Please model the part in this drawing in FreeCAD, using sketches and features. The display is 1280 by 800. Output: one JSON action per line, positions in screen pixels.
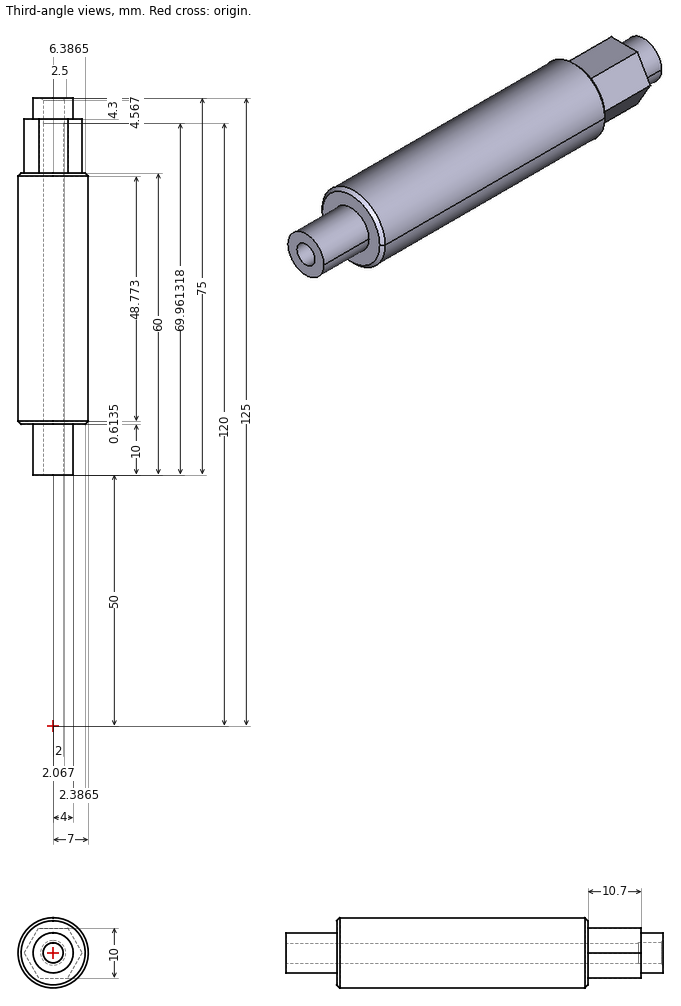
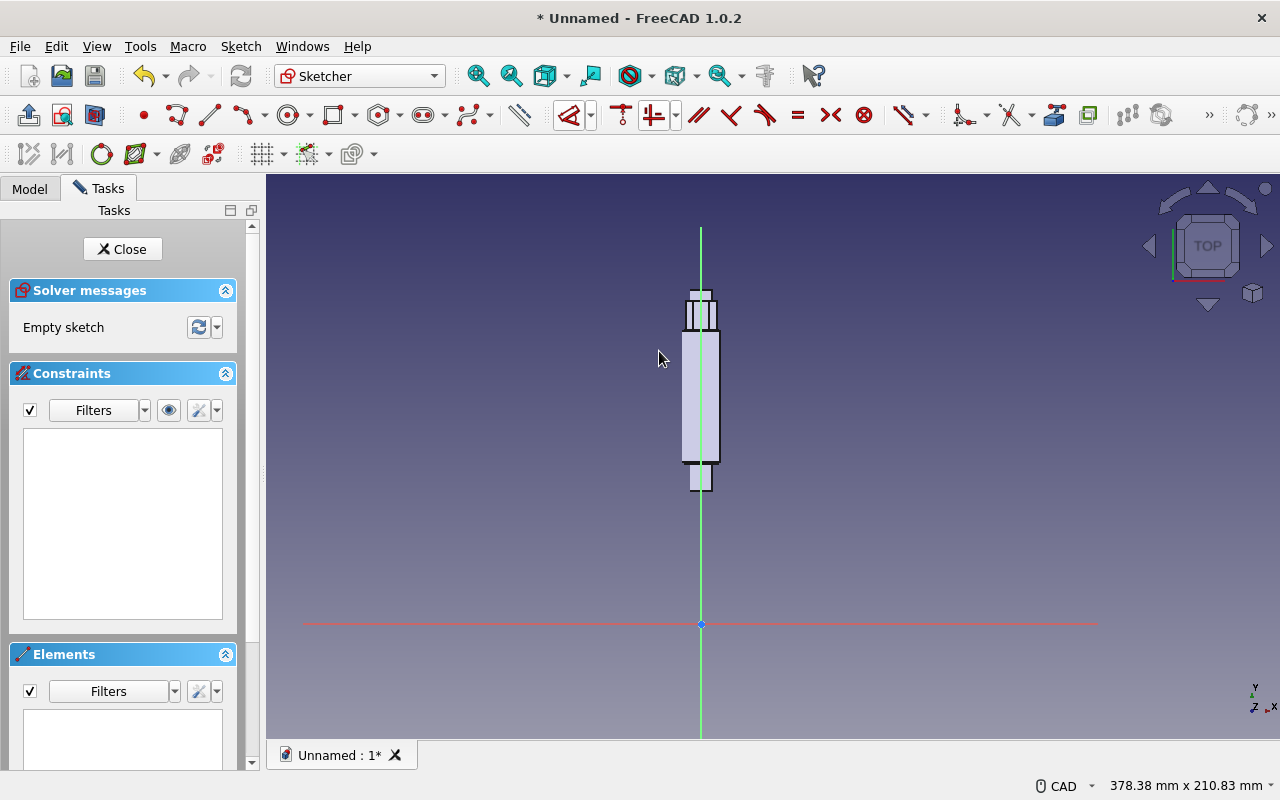
{"action": "left_click", "coordinate": [177, 116]}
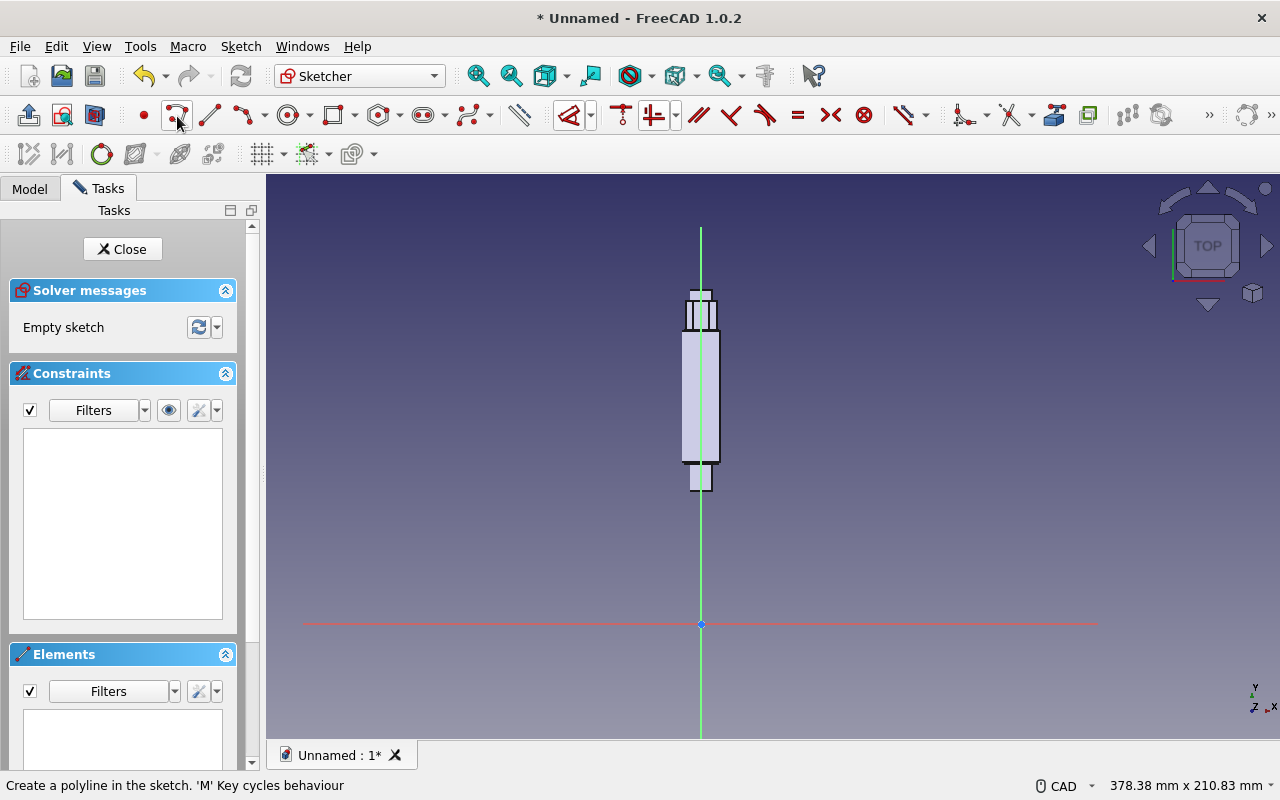
{"action": "left_click", "coordinate": [701, 491]}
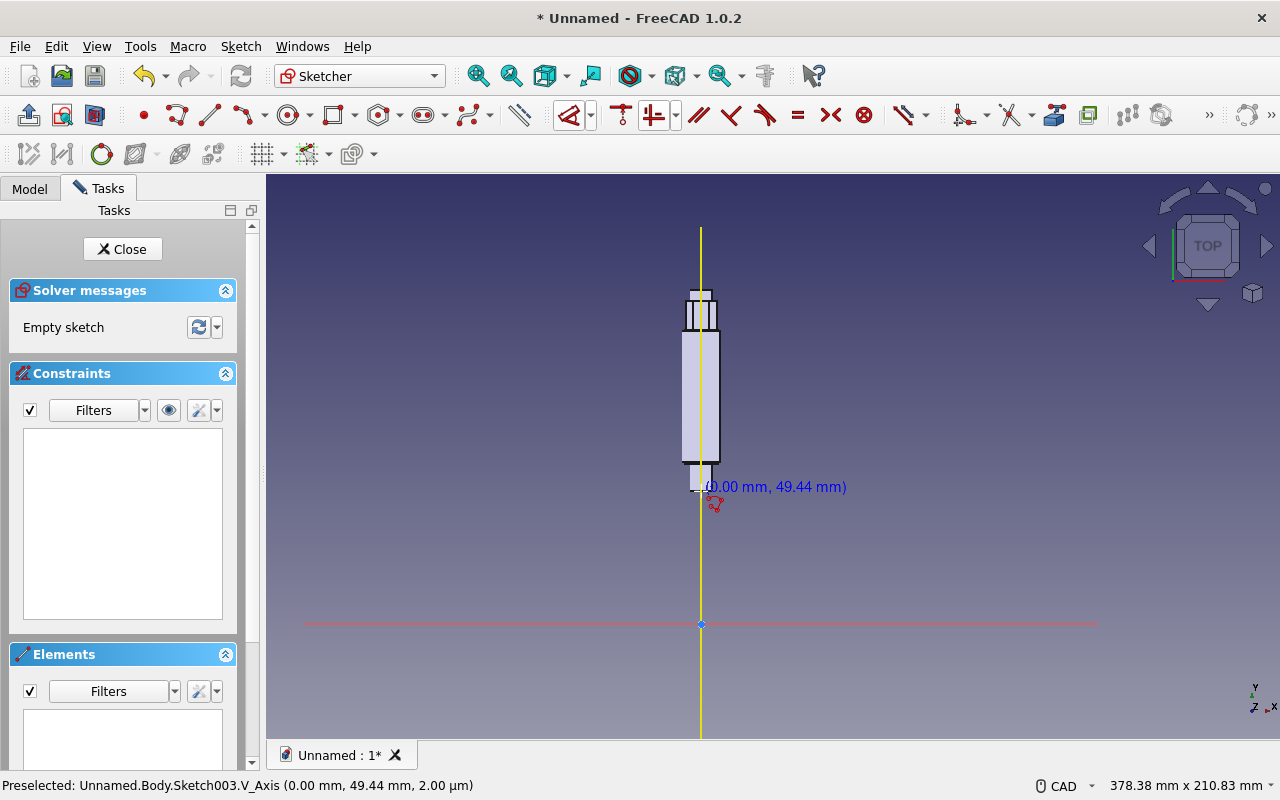
{"action": "scroll", "coordinate": [707, 491], "scroll_direction": "up", "scroll_amount": 6}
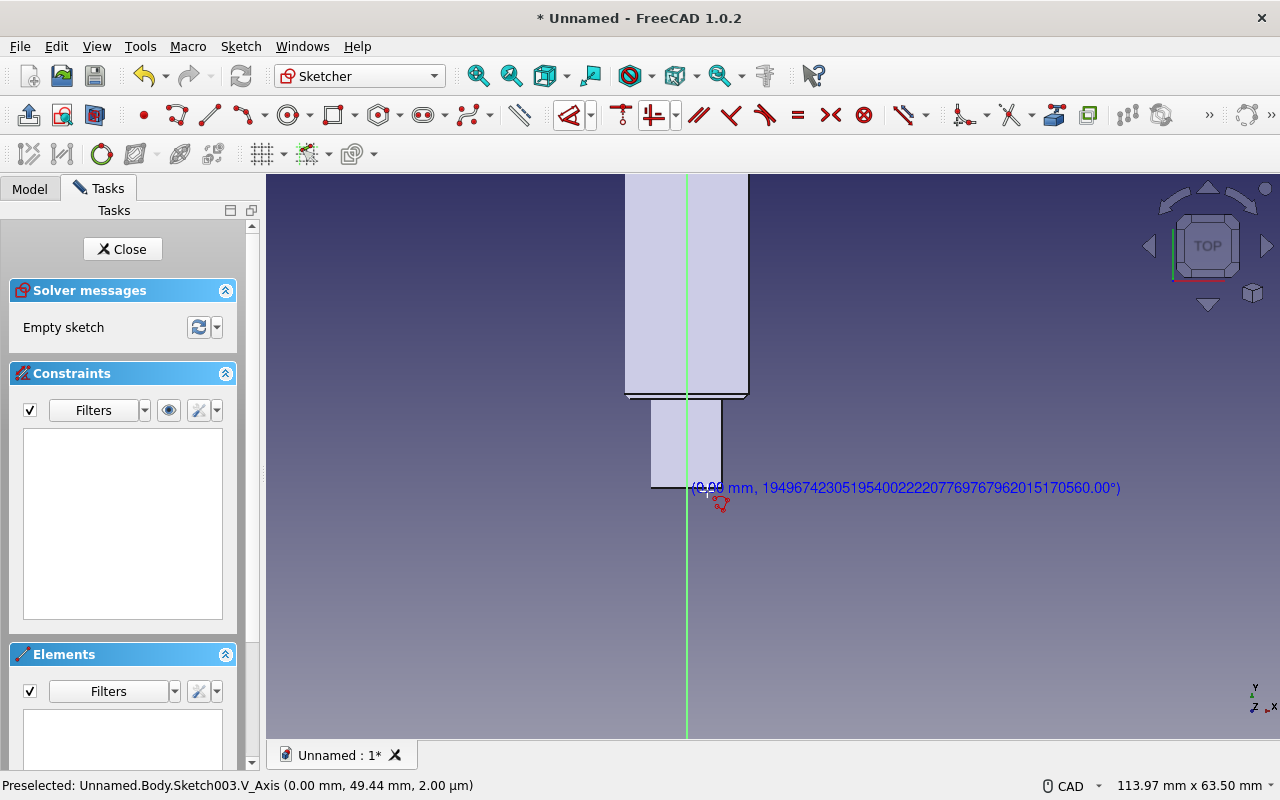
{"action": "left_click", "coordinate": [704, 490]}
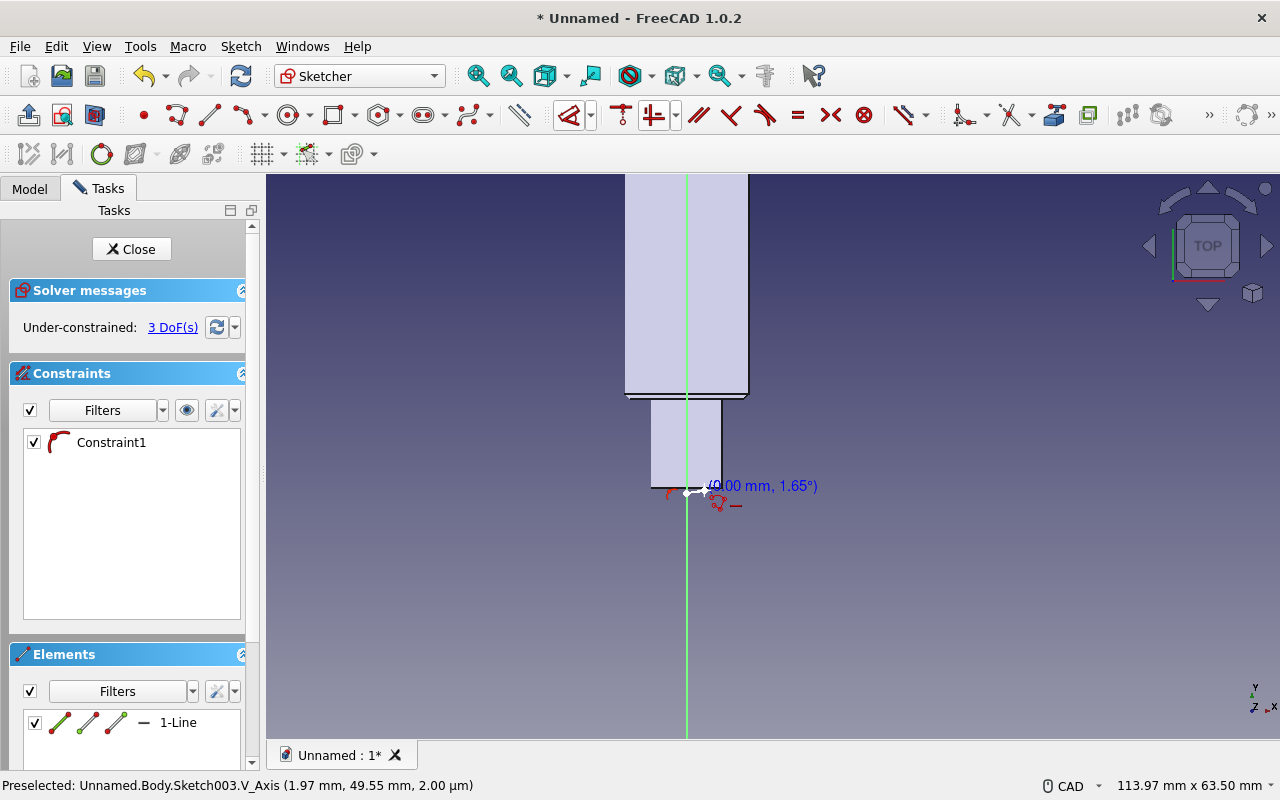
{"action": "scroll", "coordinate": [707, 491], "scroll_direction": "down", "scroll_amount": 6}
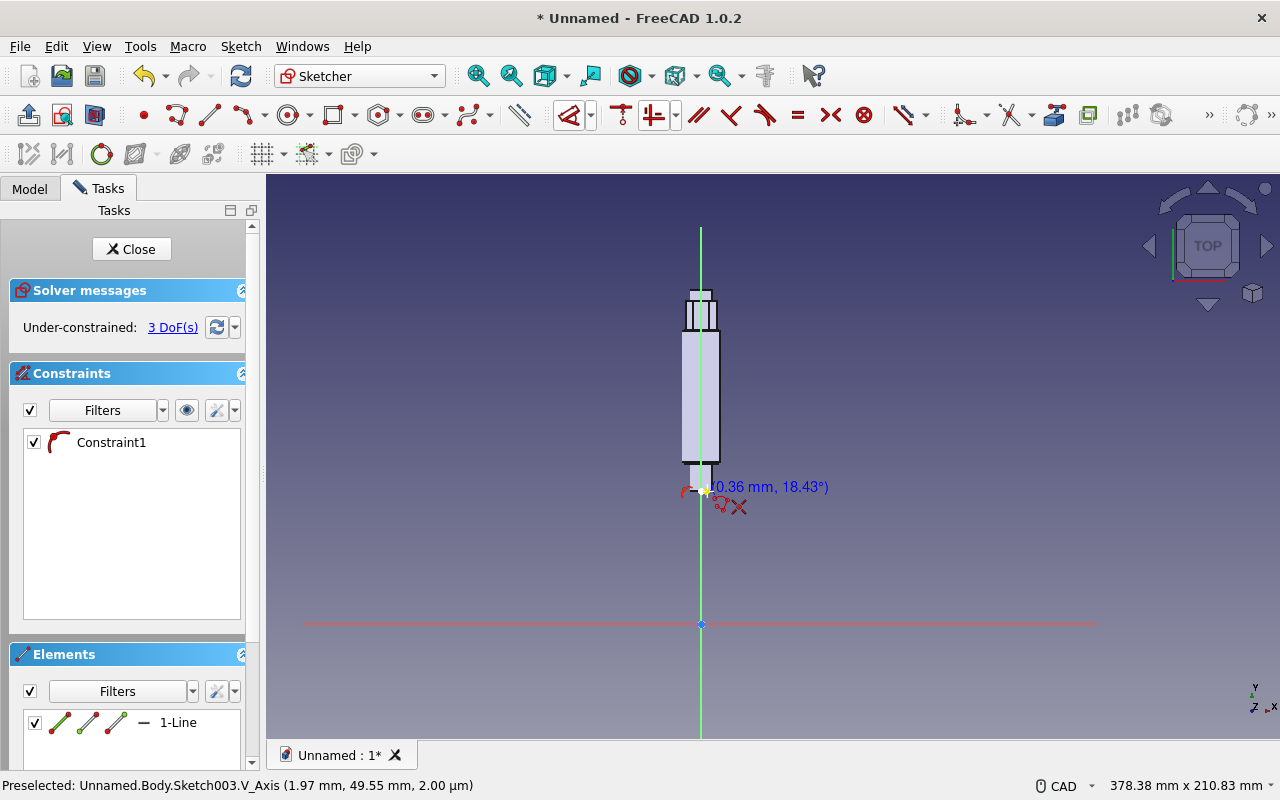
{"action": "scroll", "coordinate": [707, 303], "scroll_direction": "up", "scroll_amount": 6}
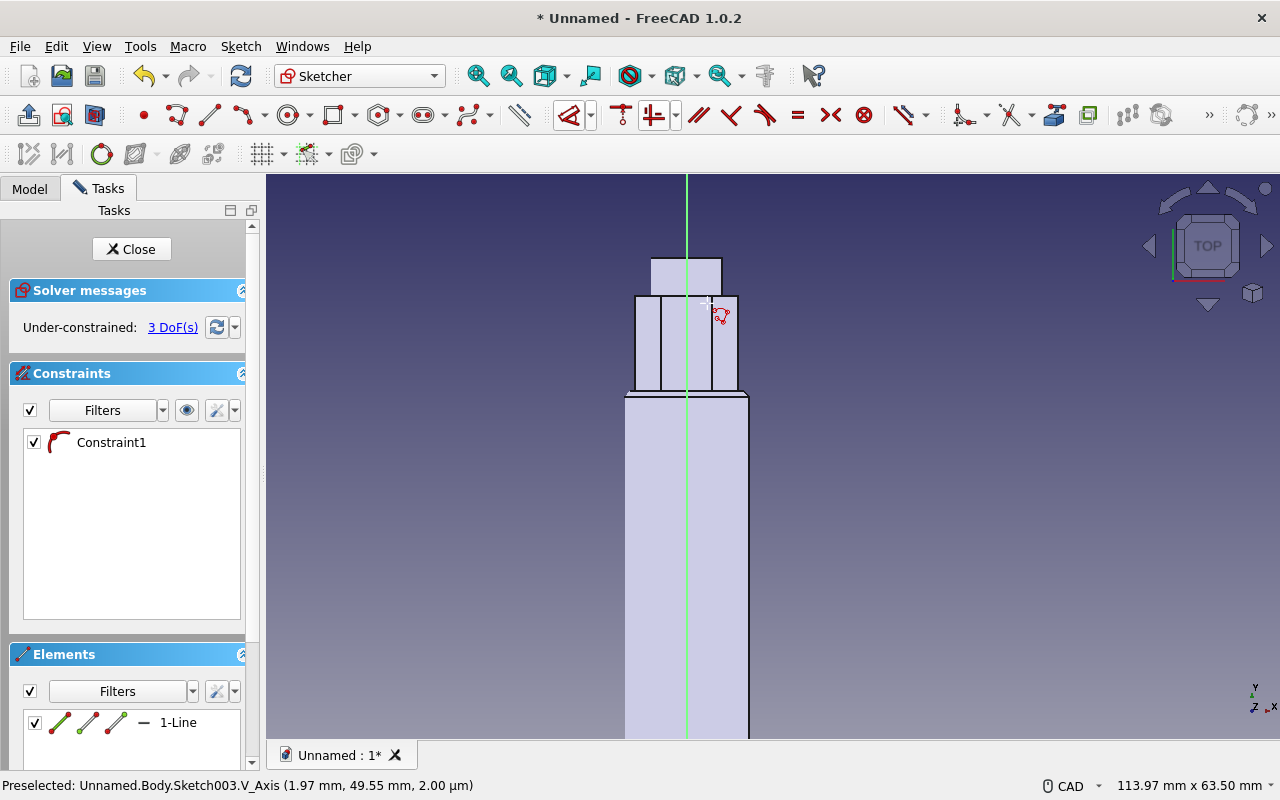
{"action": "left_click", "coordinate": [704, 303]}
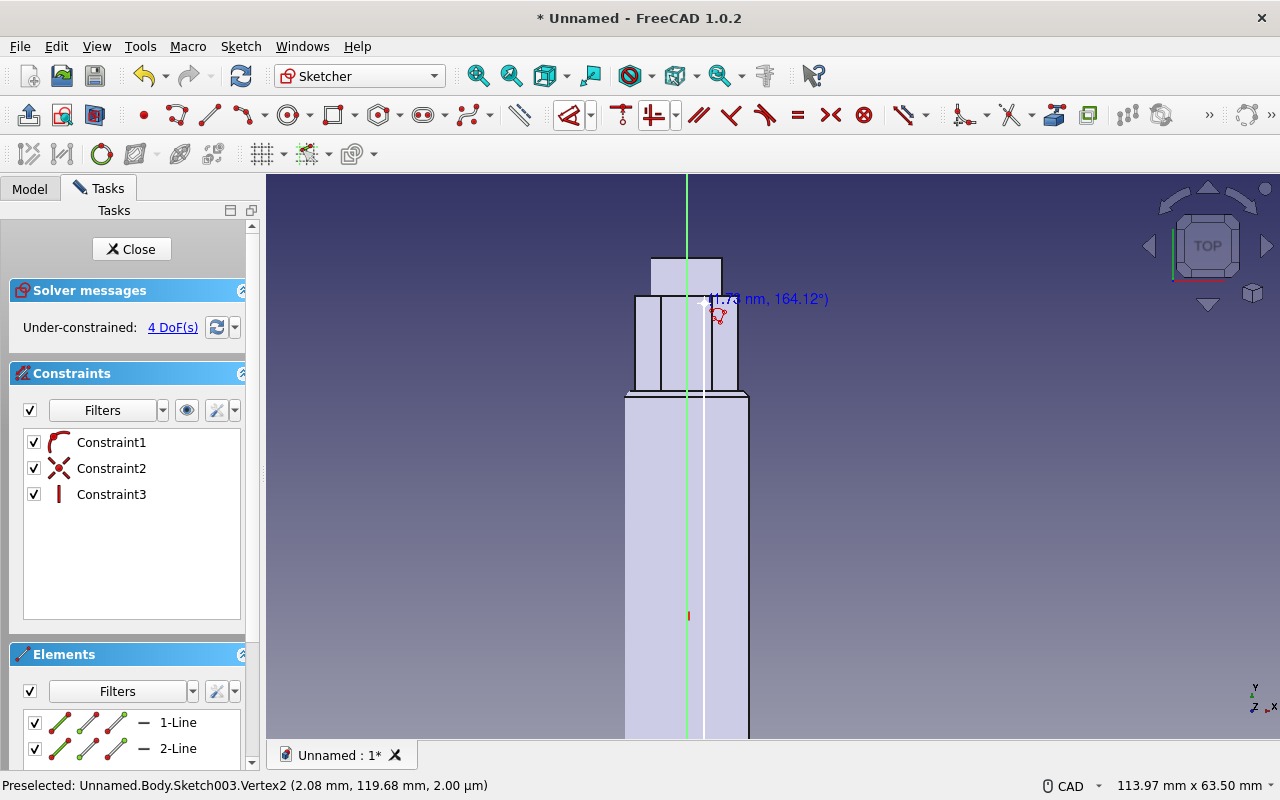
{"action": "scroll", "coordinate": [705, 302], "scroll_direction": "up", "scroll_amount": 16}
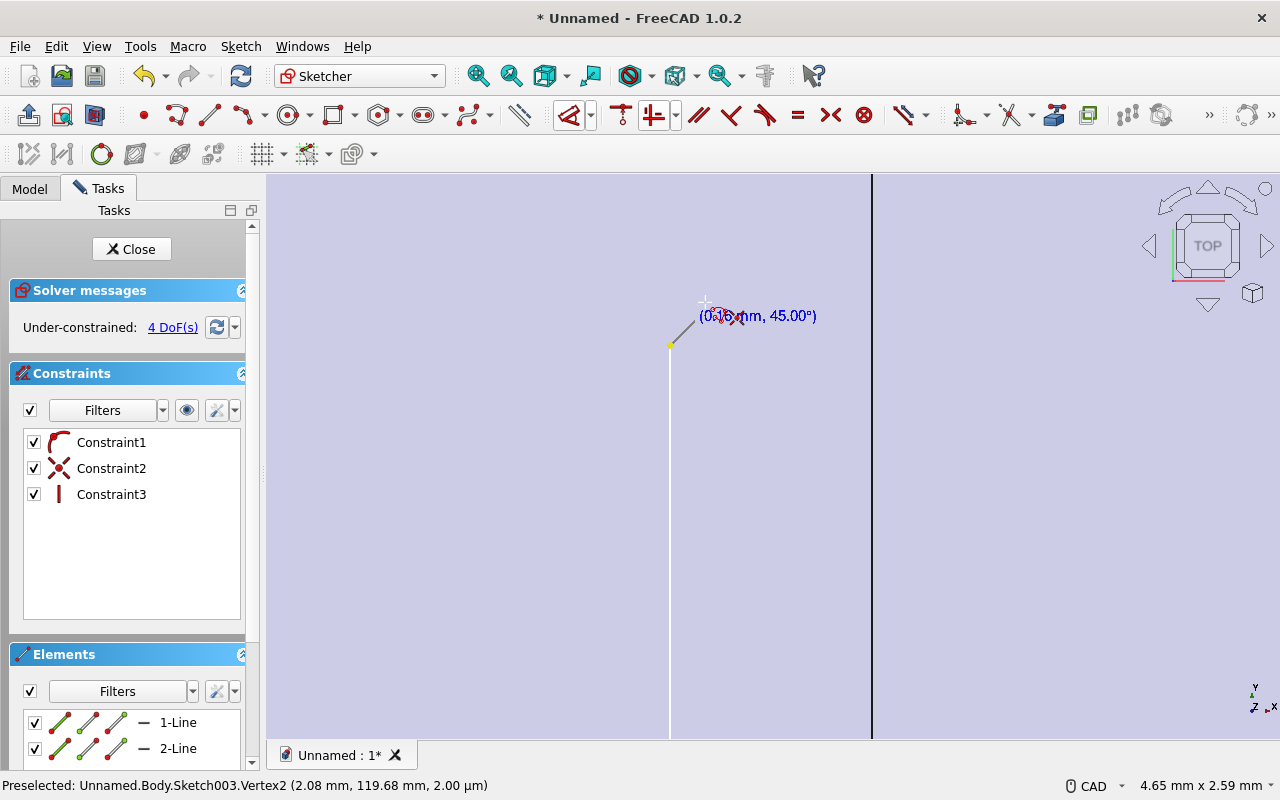
{"action": "left_click", "coordinate": [693, 301]}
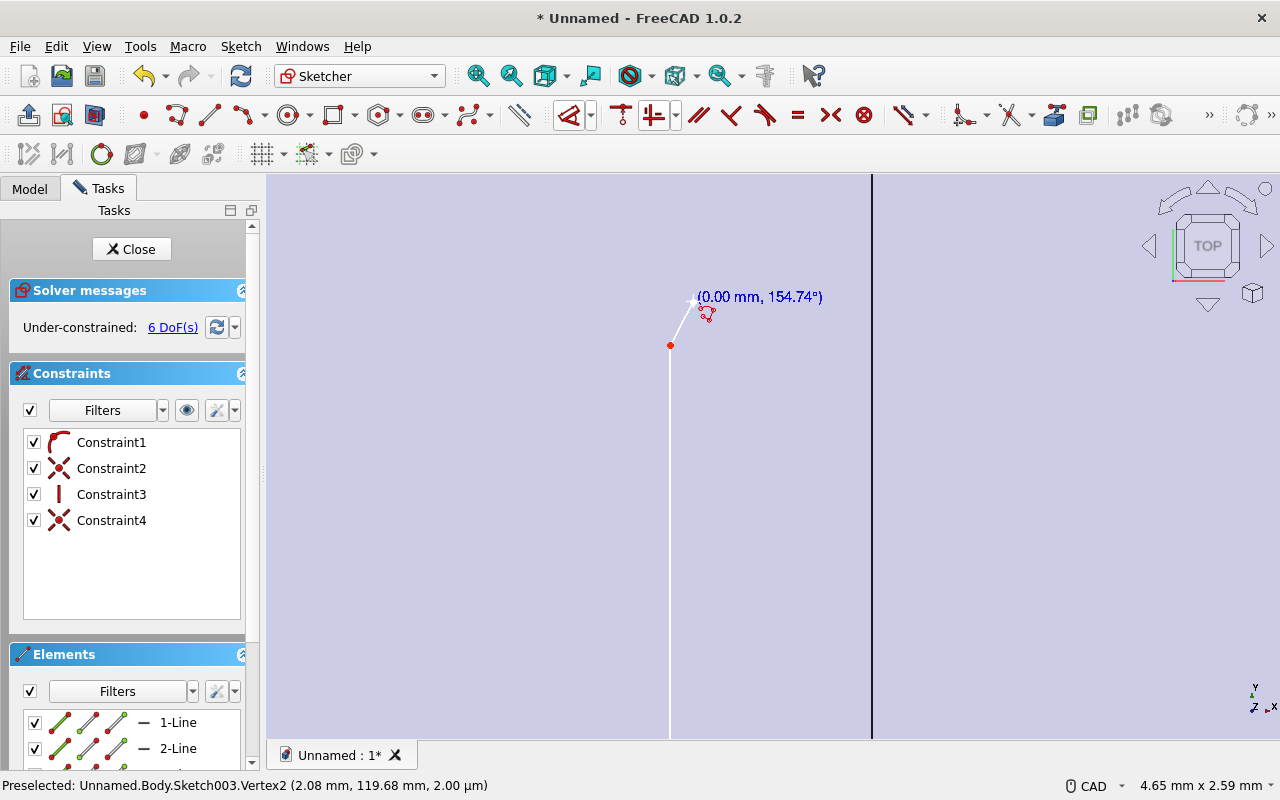
{"action": "scroll", "coordinate": [704, 456], "scroll_direction": "down", "scroll_amount": 15}